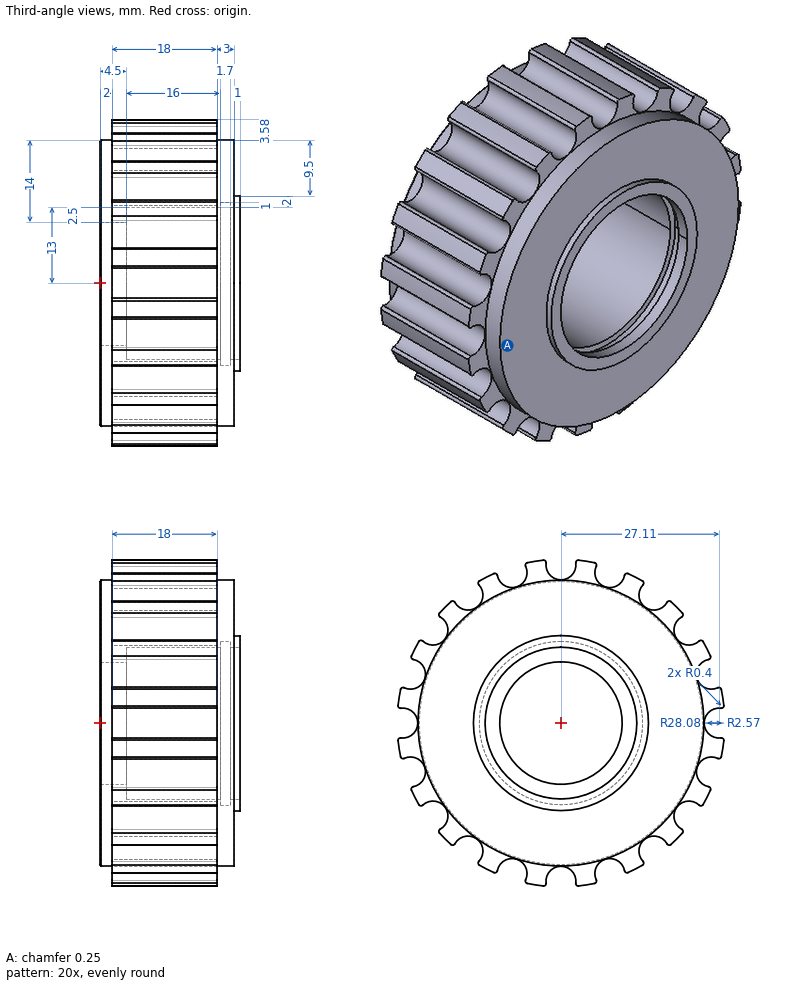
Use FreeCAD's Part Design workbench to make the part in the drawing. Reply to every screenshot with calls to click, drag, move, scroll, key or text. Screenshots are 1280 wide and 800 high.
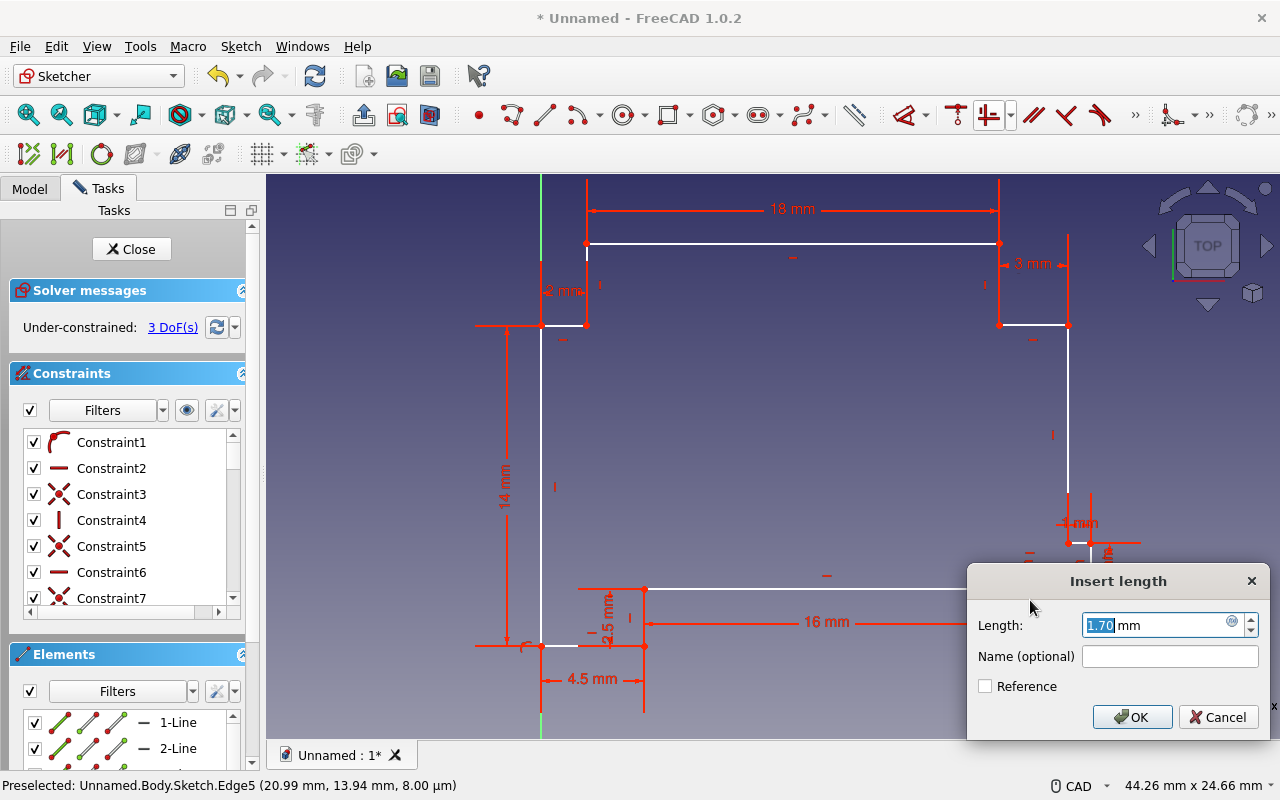
text(1.7)
key(Return)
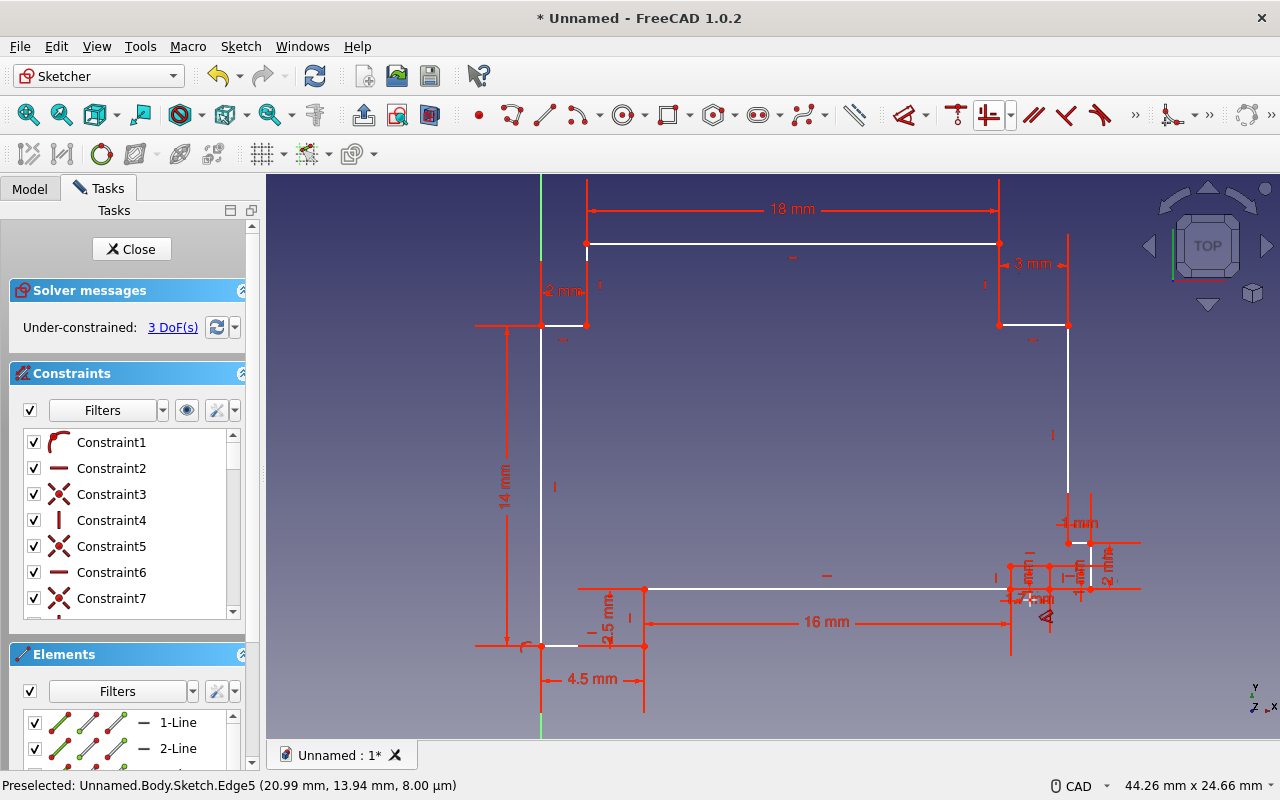
click(1068, 478)
click(1102, 434)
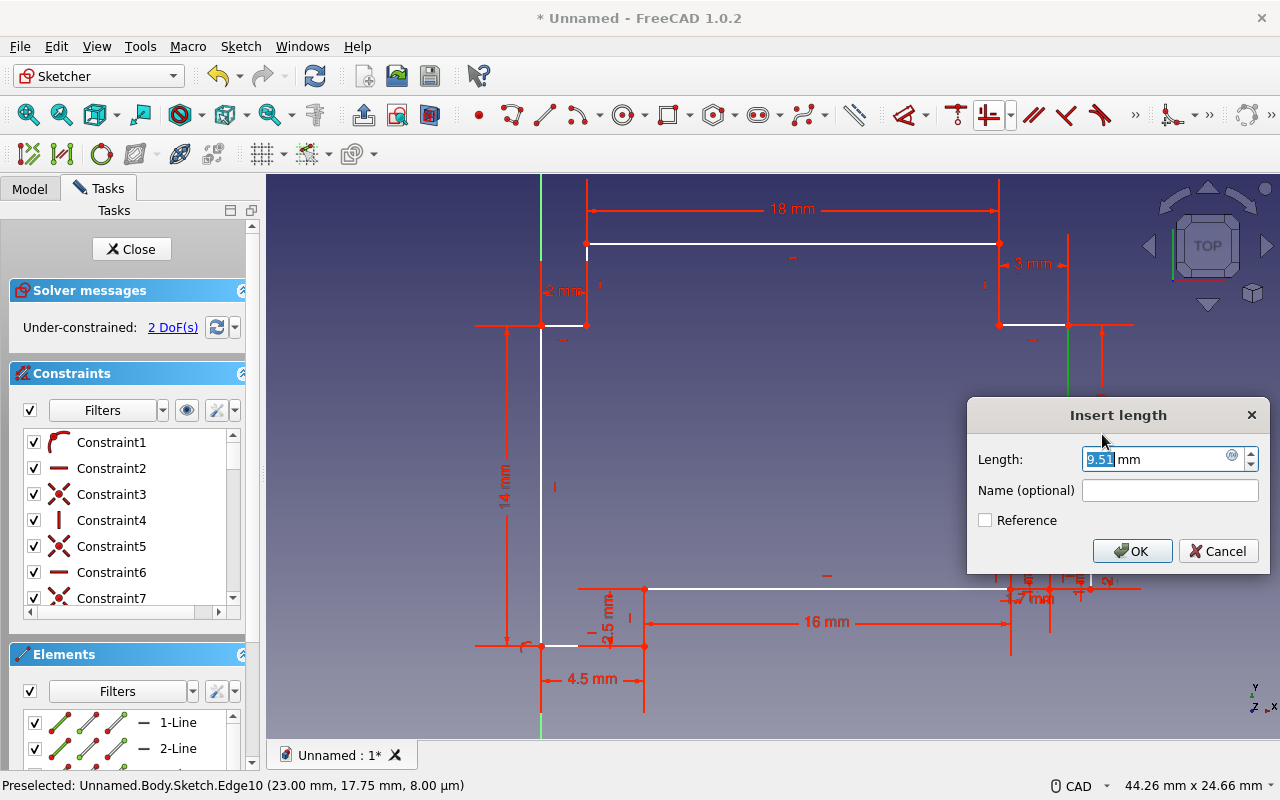
text(9.5)
key(Return)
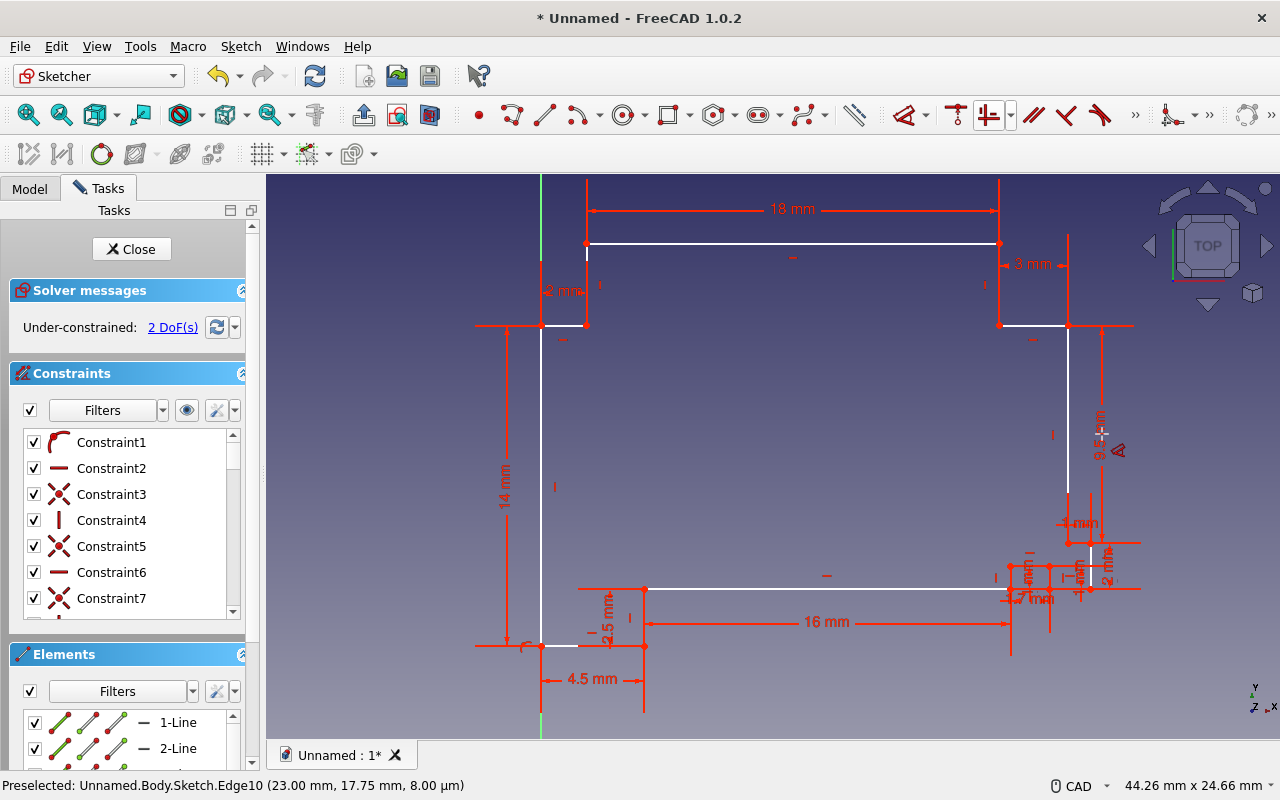
click(644, 589)
click(507, 650)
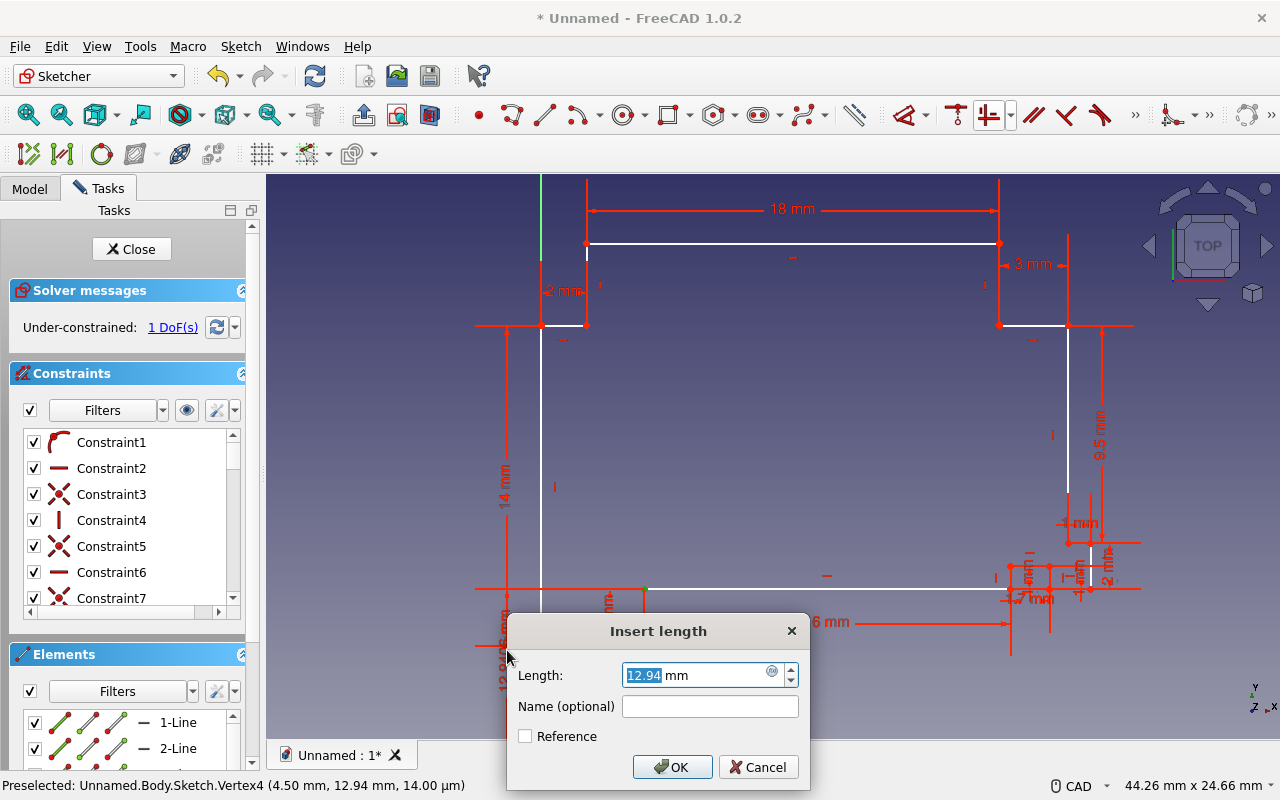
text(13)
key(Return)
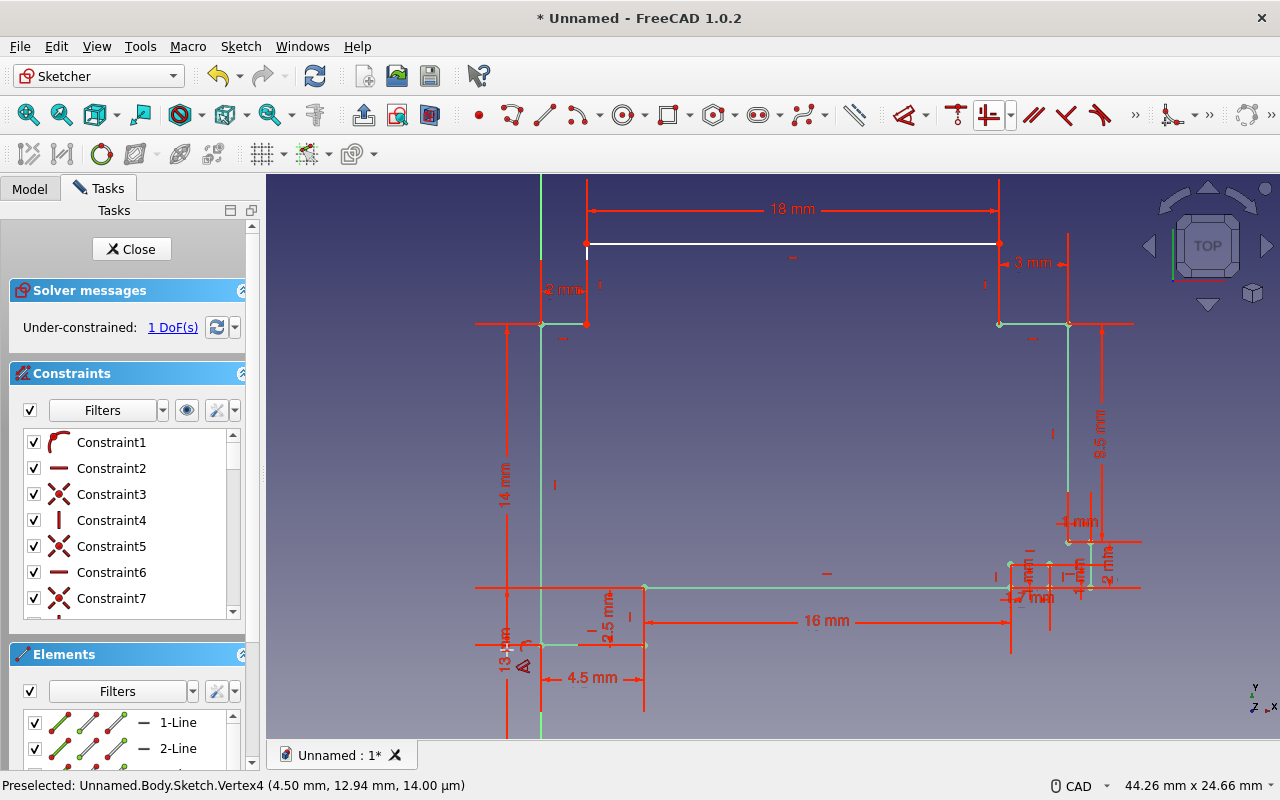
click(999, 300)
click(1033, 284)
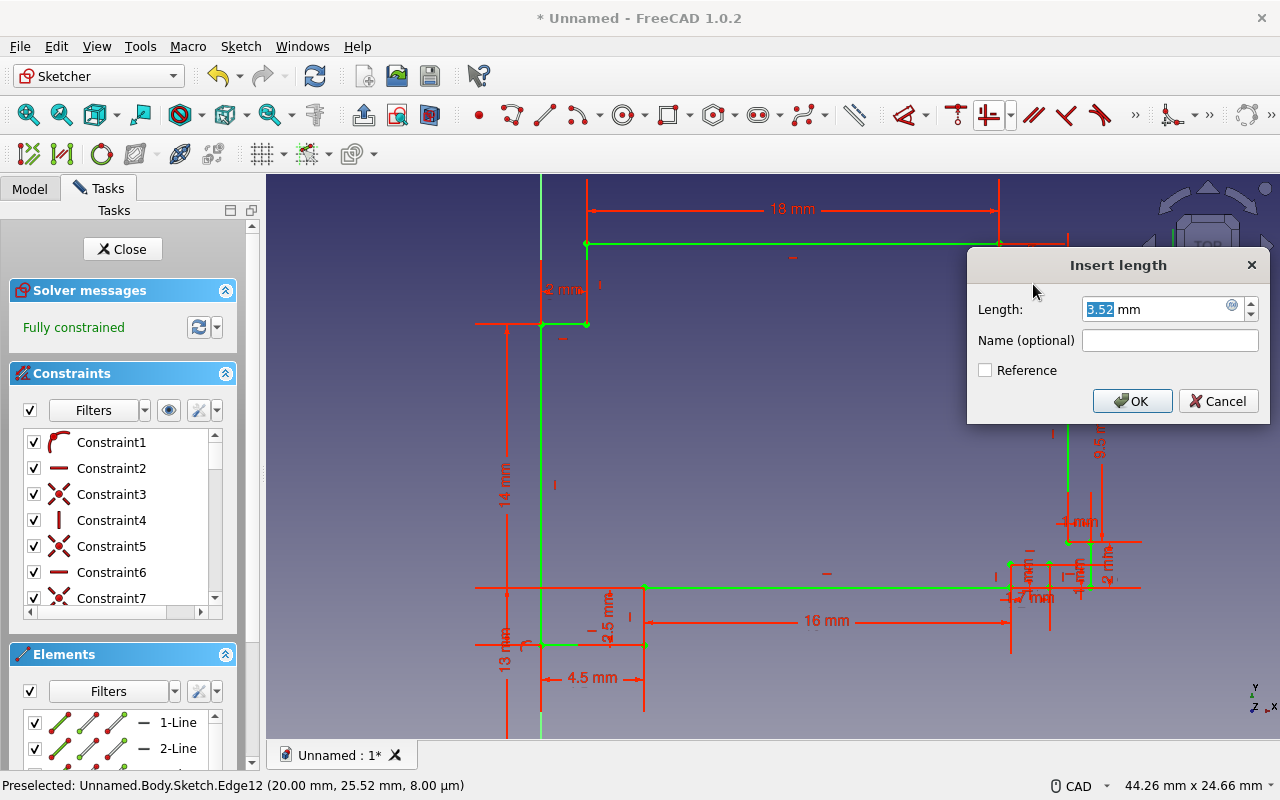
text(3.58)
key(Return)
key(Escape)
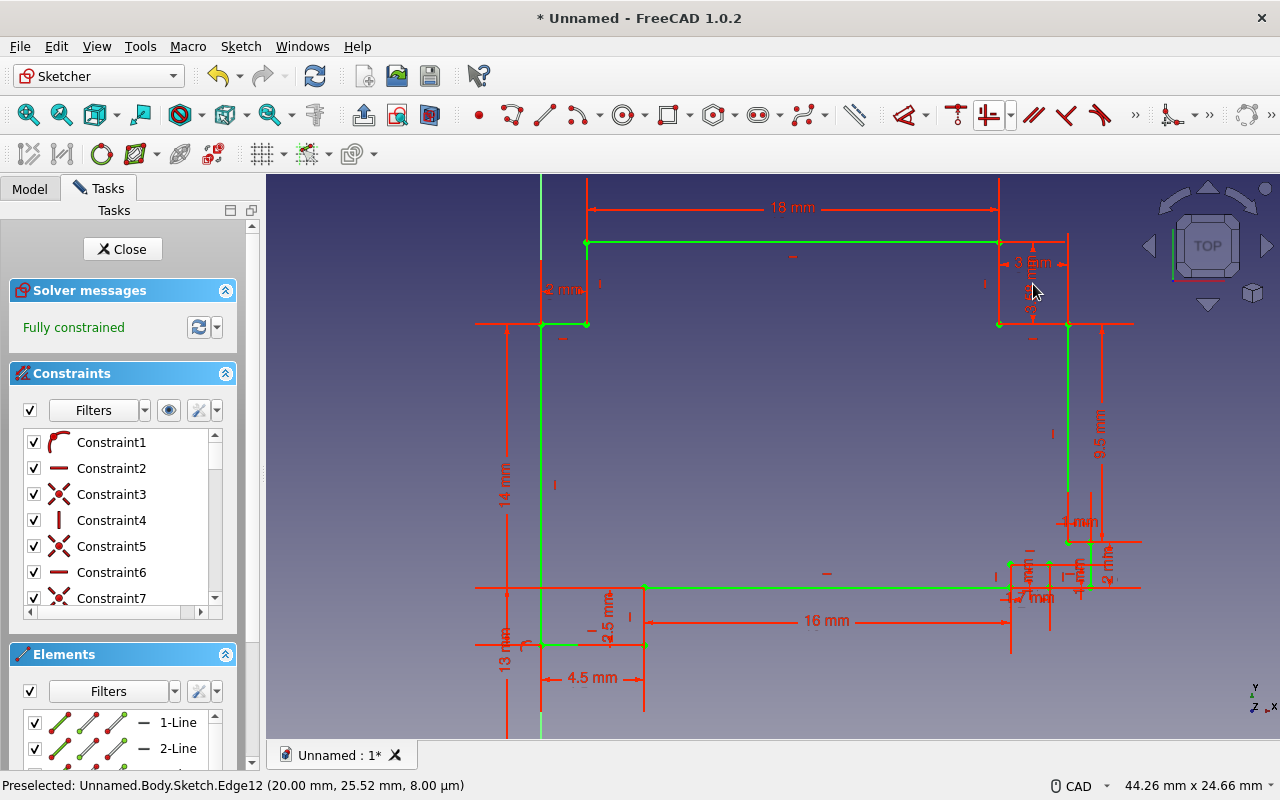
click(123, 249)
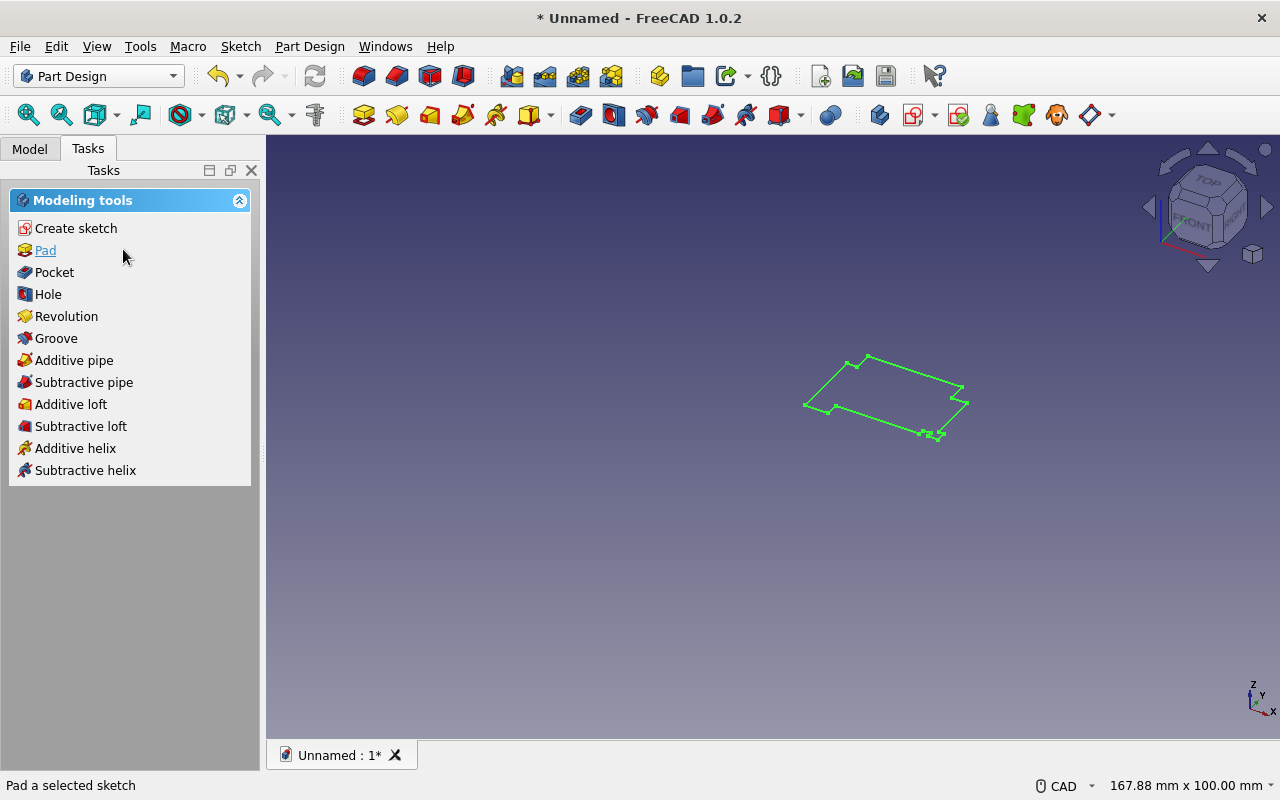
click(397, 116)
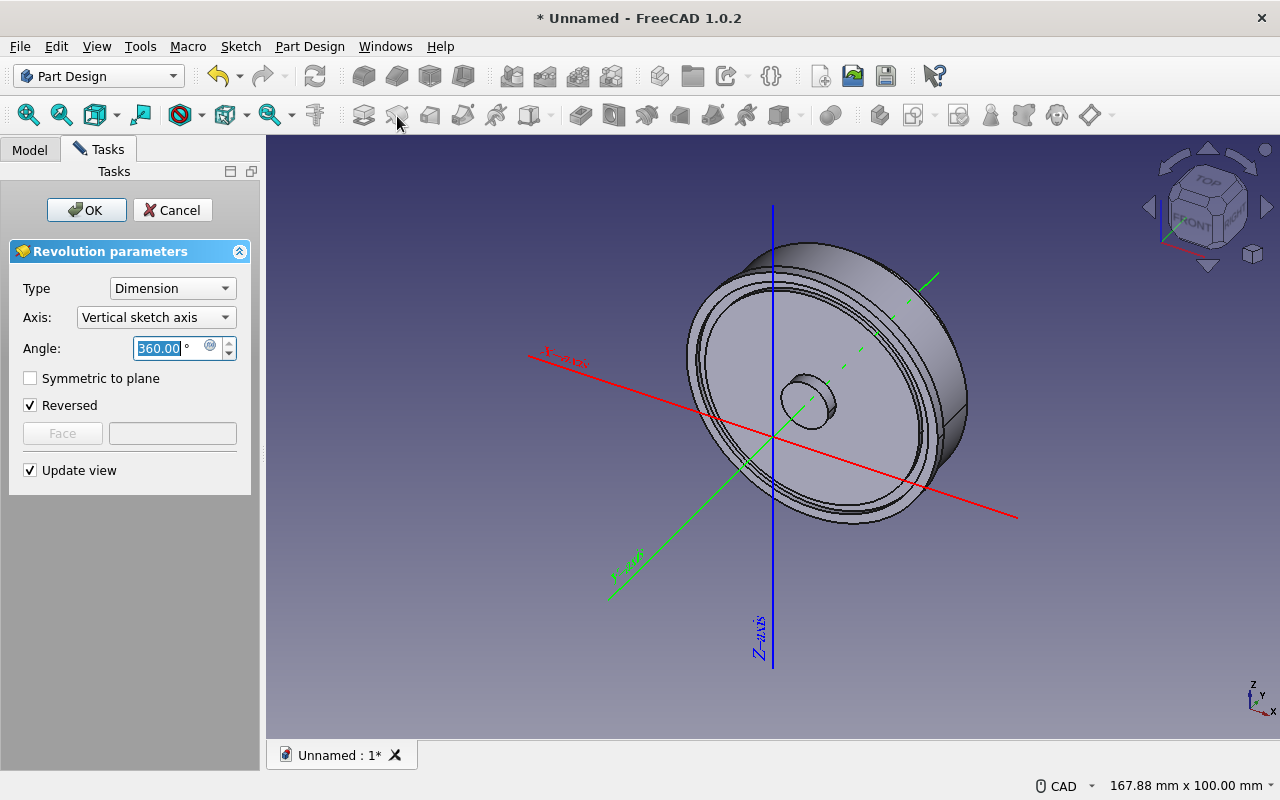
click(157, 318)